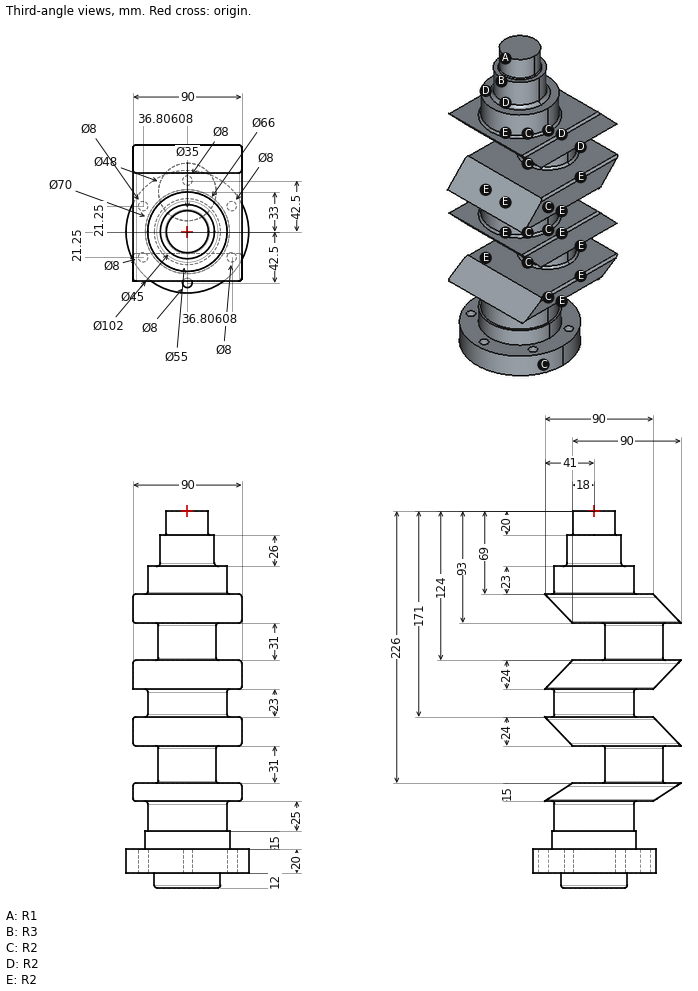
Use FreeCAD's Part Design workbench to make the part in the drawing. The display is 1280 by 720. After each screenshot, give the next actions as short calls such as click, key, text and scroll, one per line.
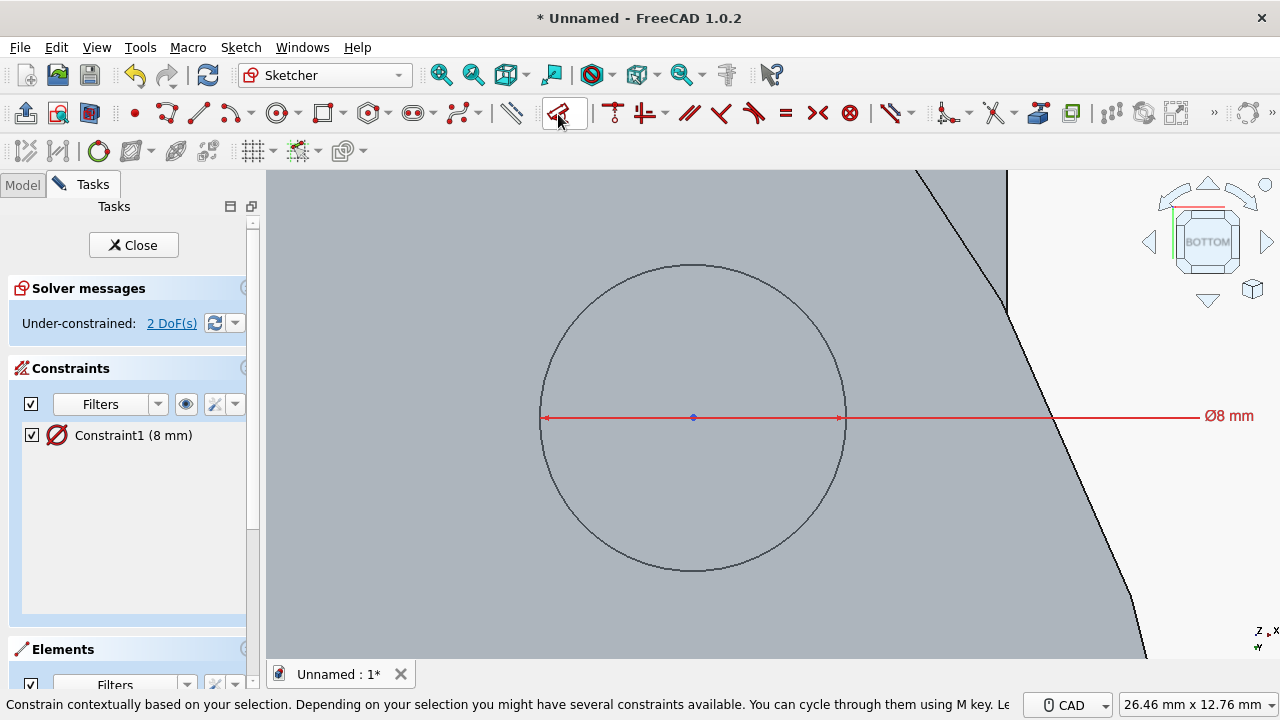
click(693, 418)
click(727, 525)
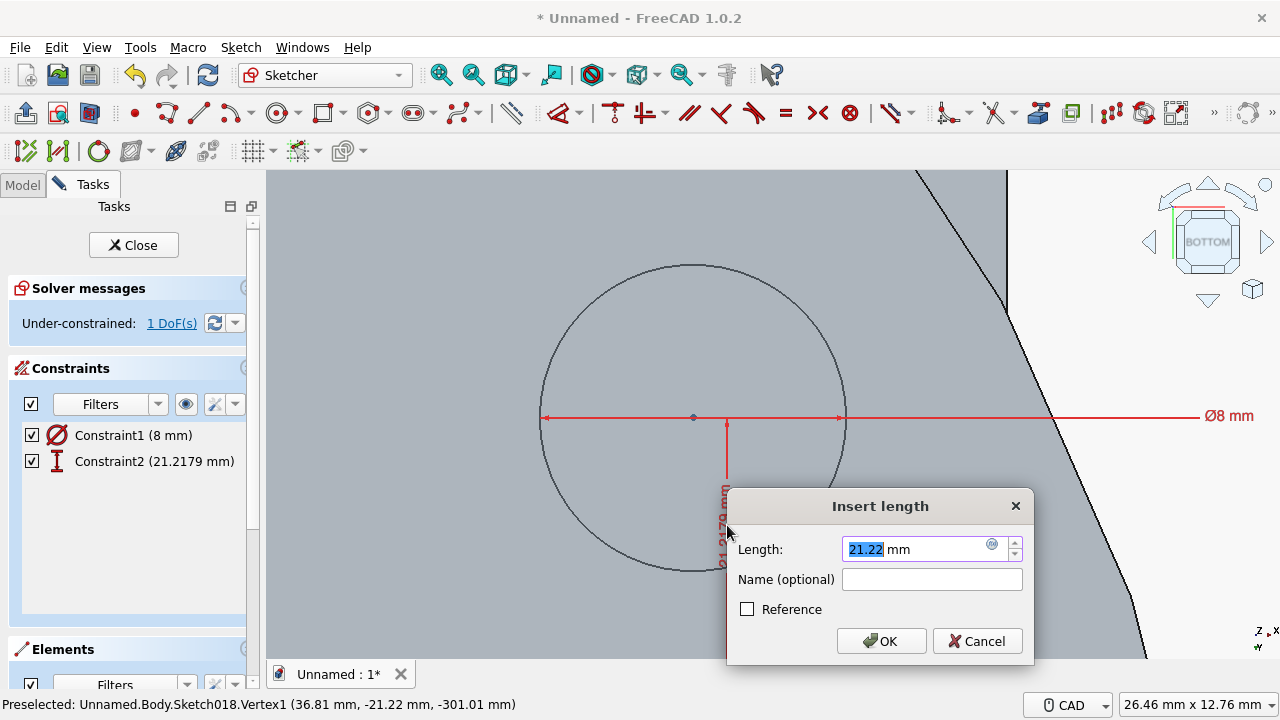
text(21.25)
key(Return)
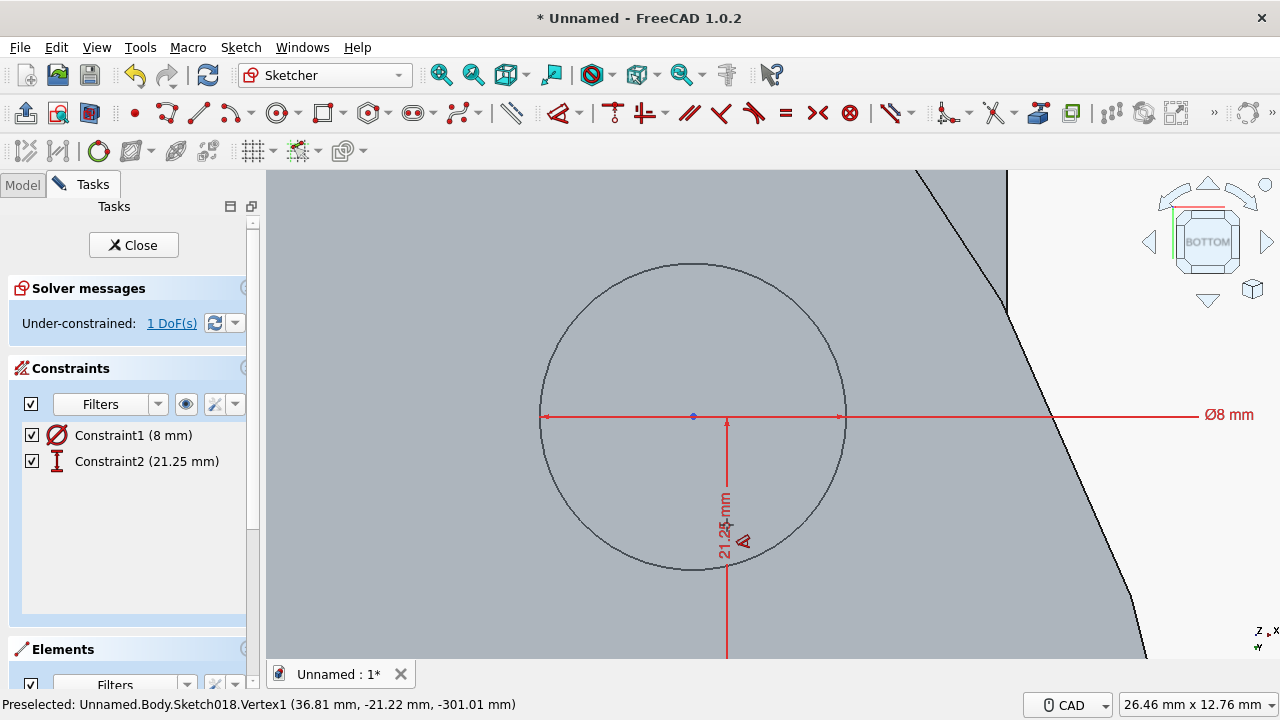
click(693, 417)
click(494, 383)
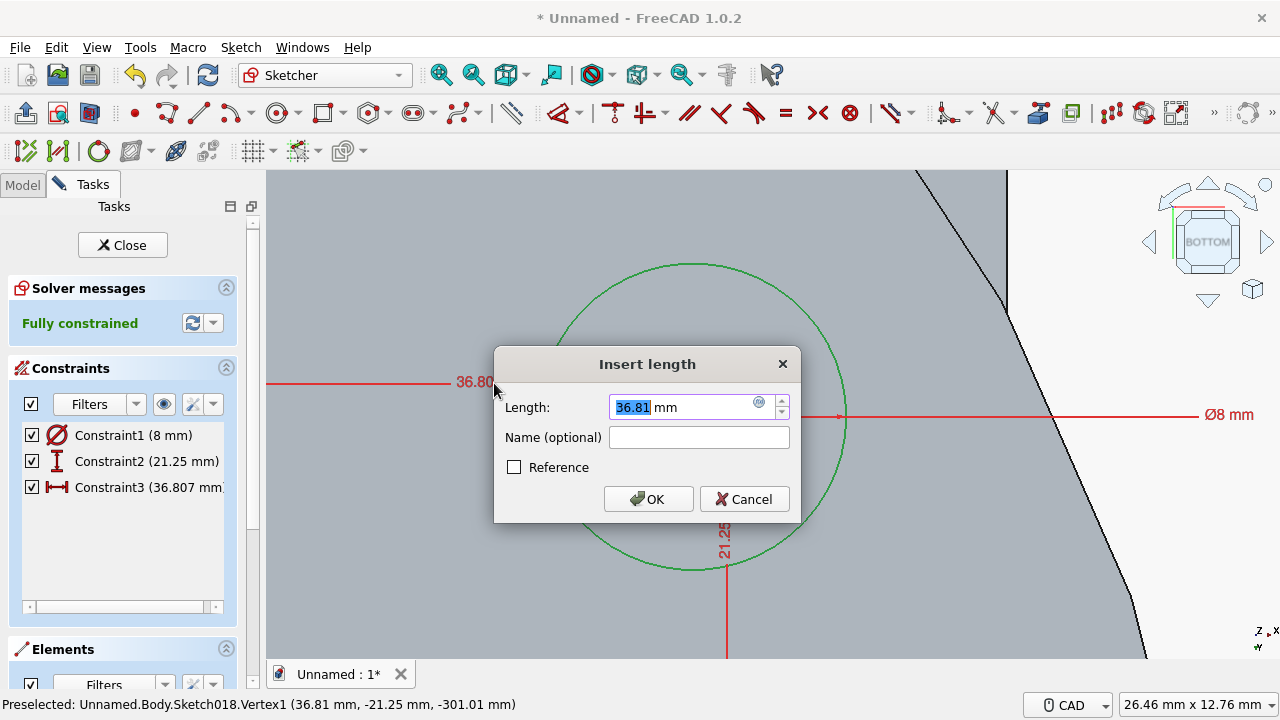
text(36.80608)
key(Return)
key(Escape)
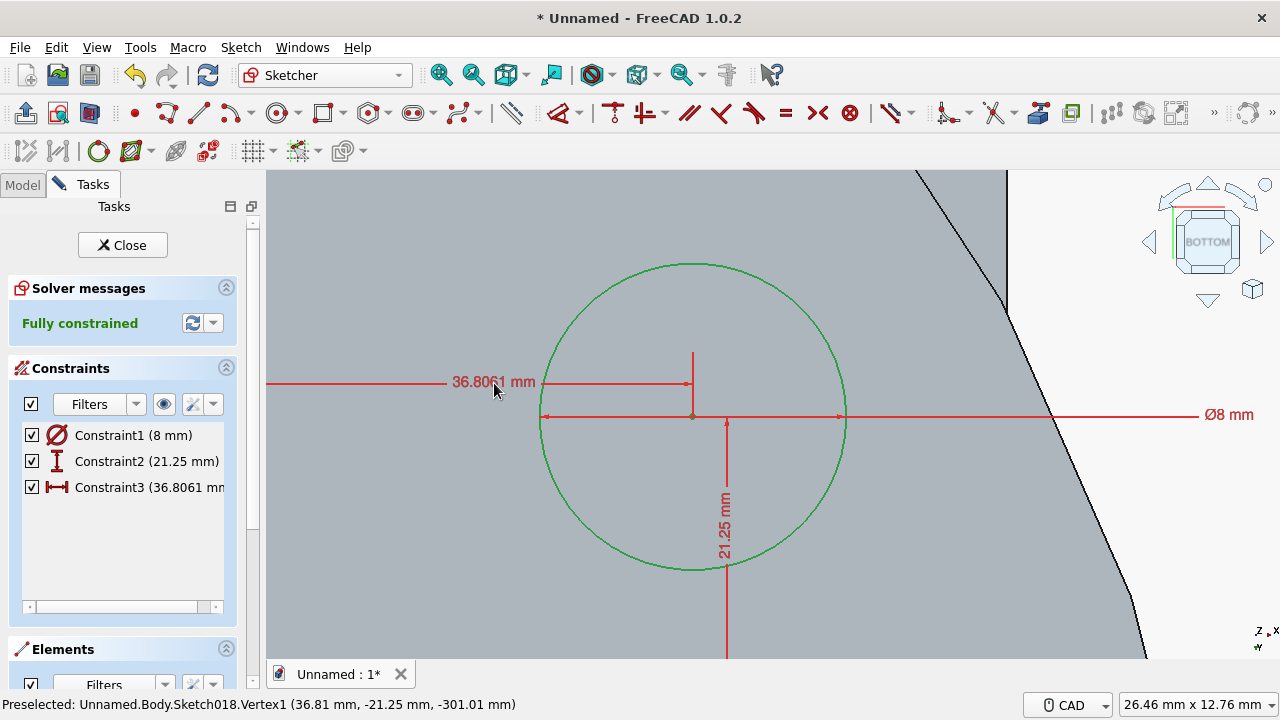
click(123, 245)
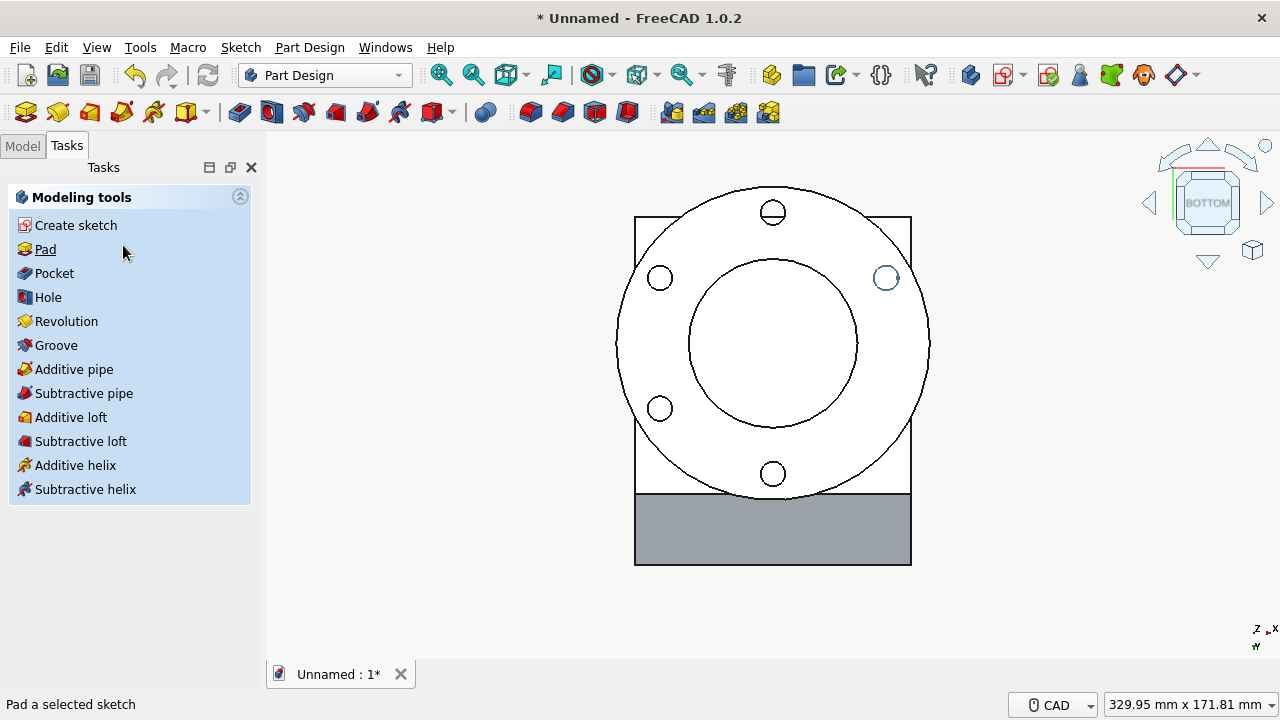
click(240, 112)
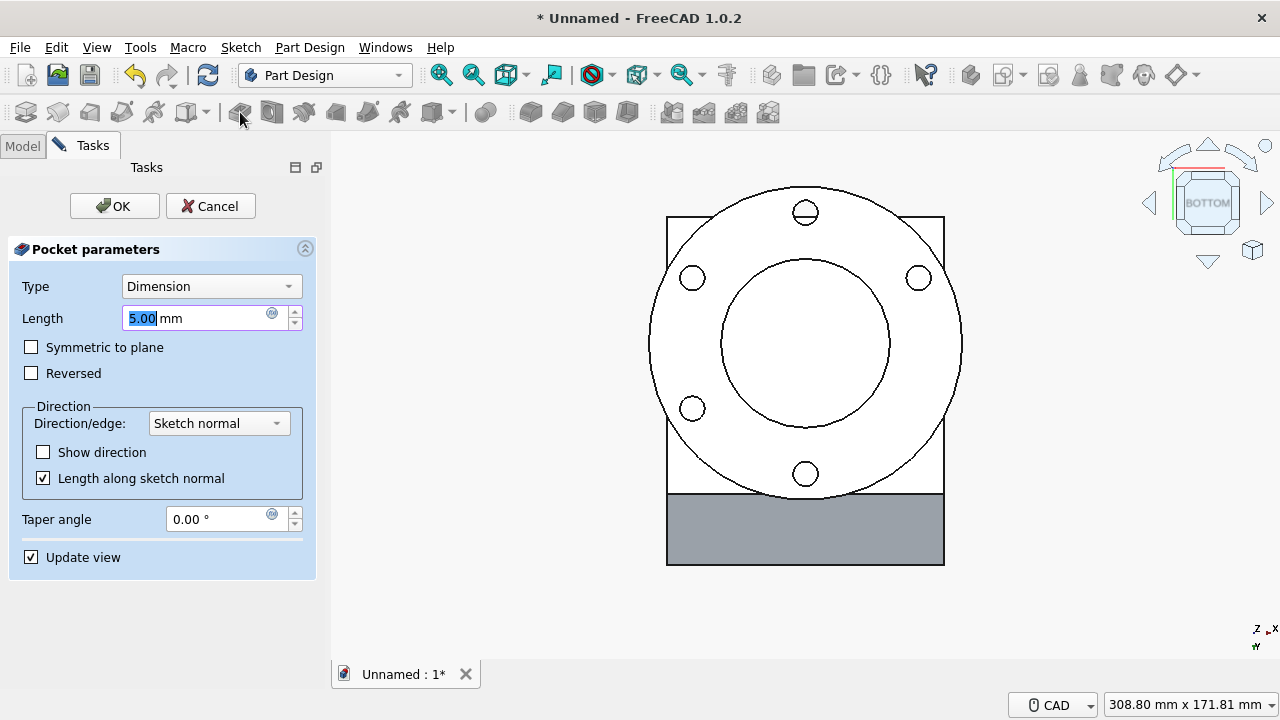
click(212, 286)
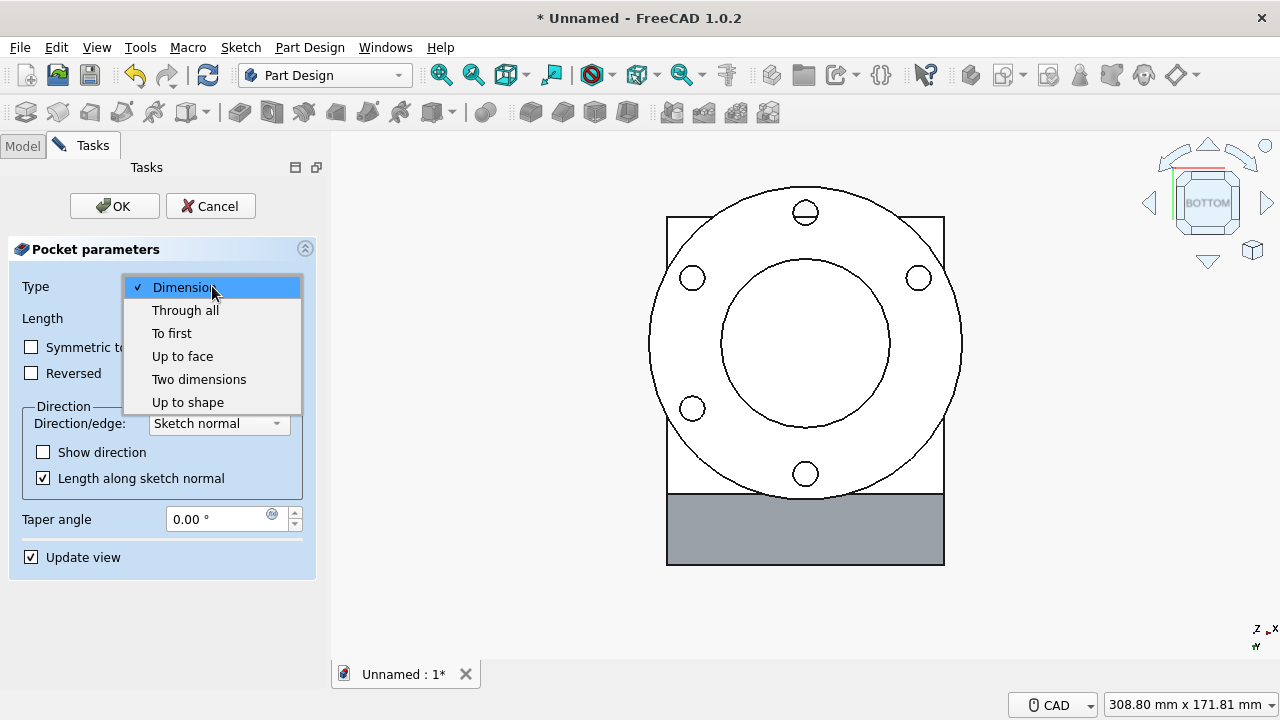
click(212, 334)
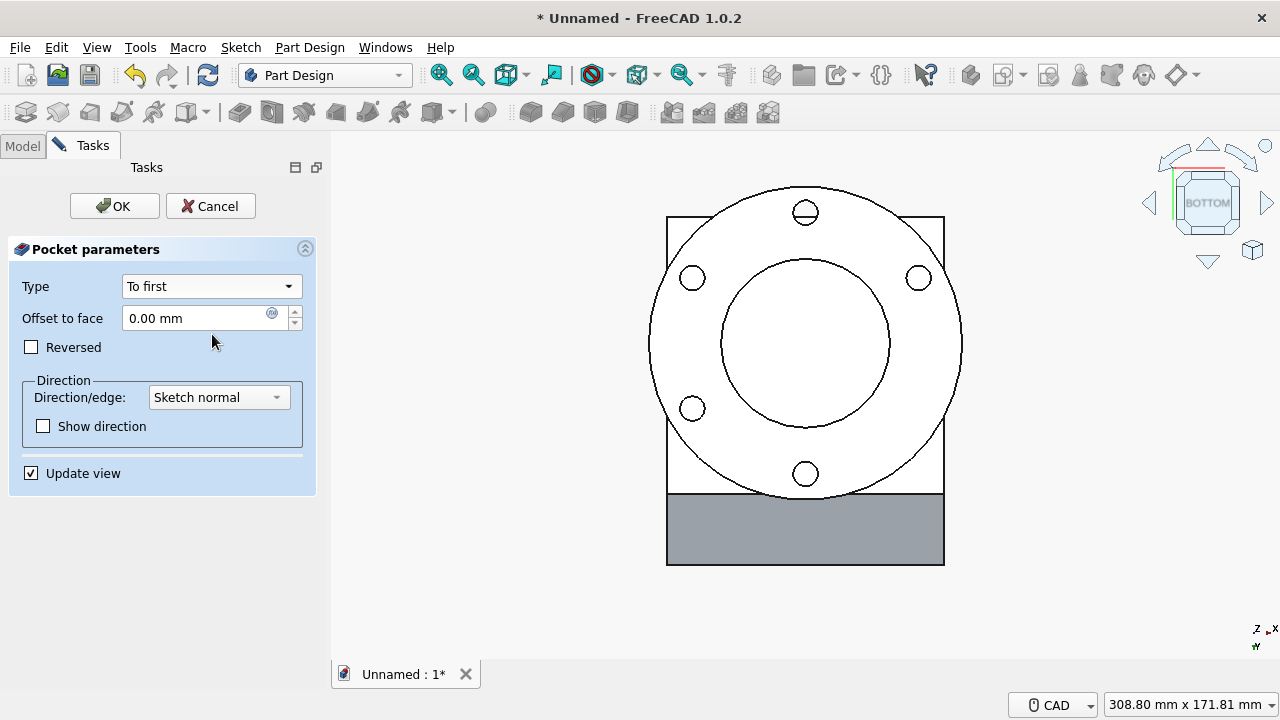
click(115, 206)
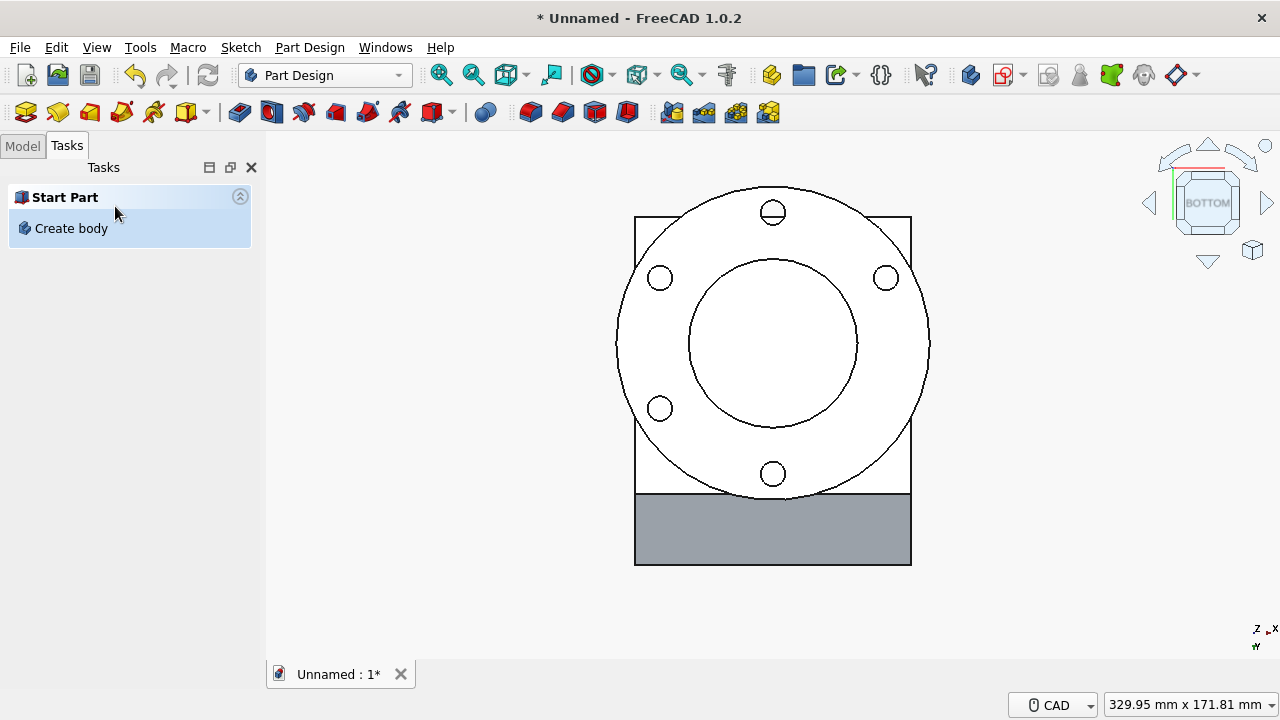
click(863, 432)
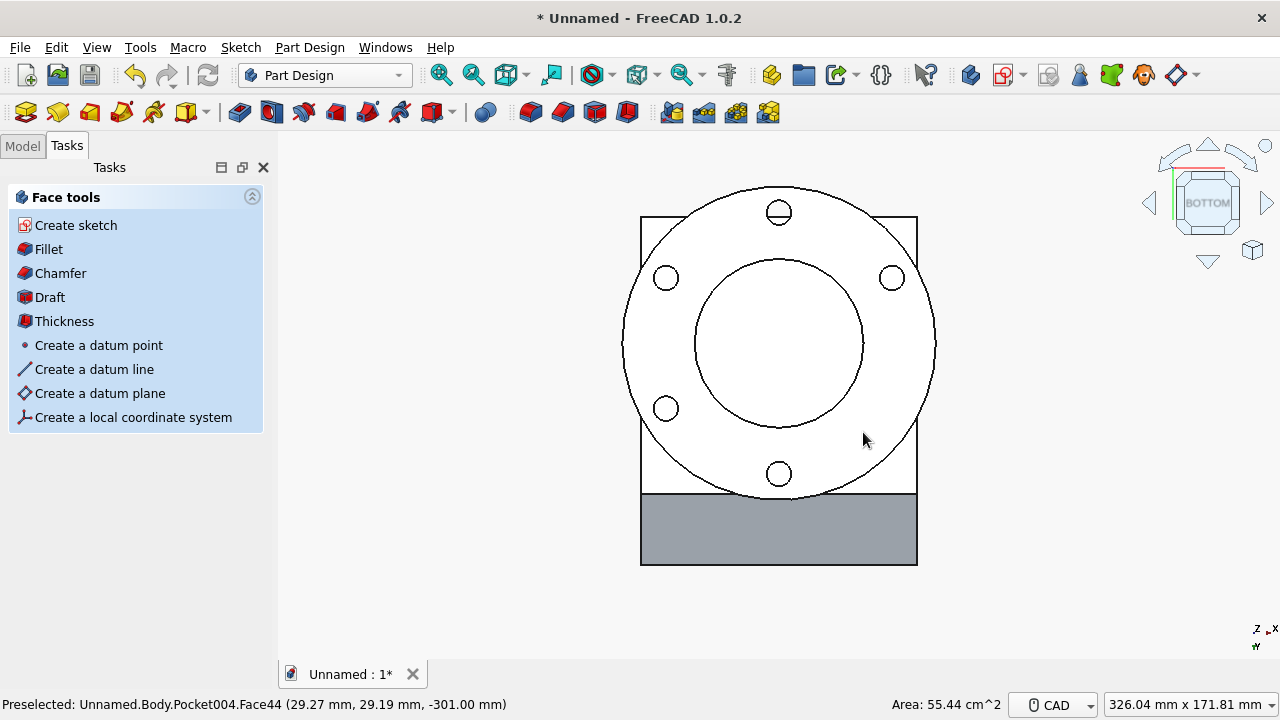
click(1004, 76)